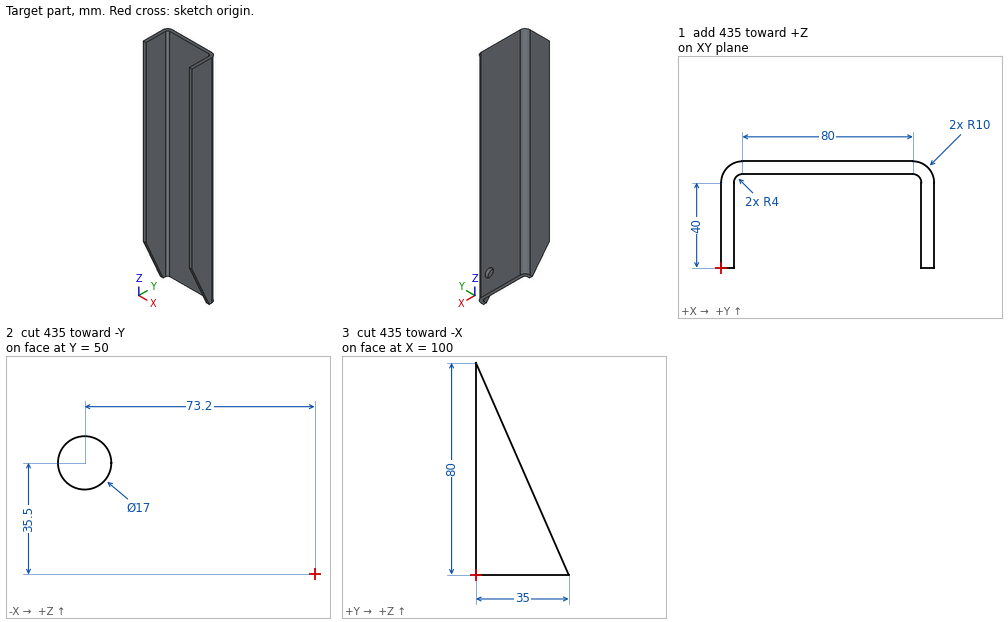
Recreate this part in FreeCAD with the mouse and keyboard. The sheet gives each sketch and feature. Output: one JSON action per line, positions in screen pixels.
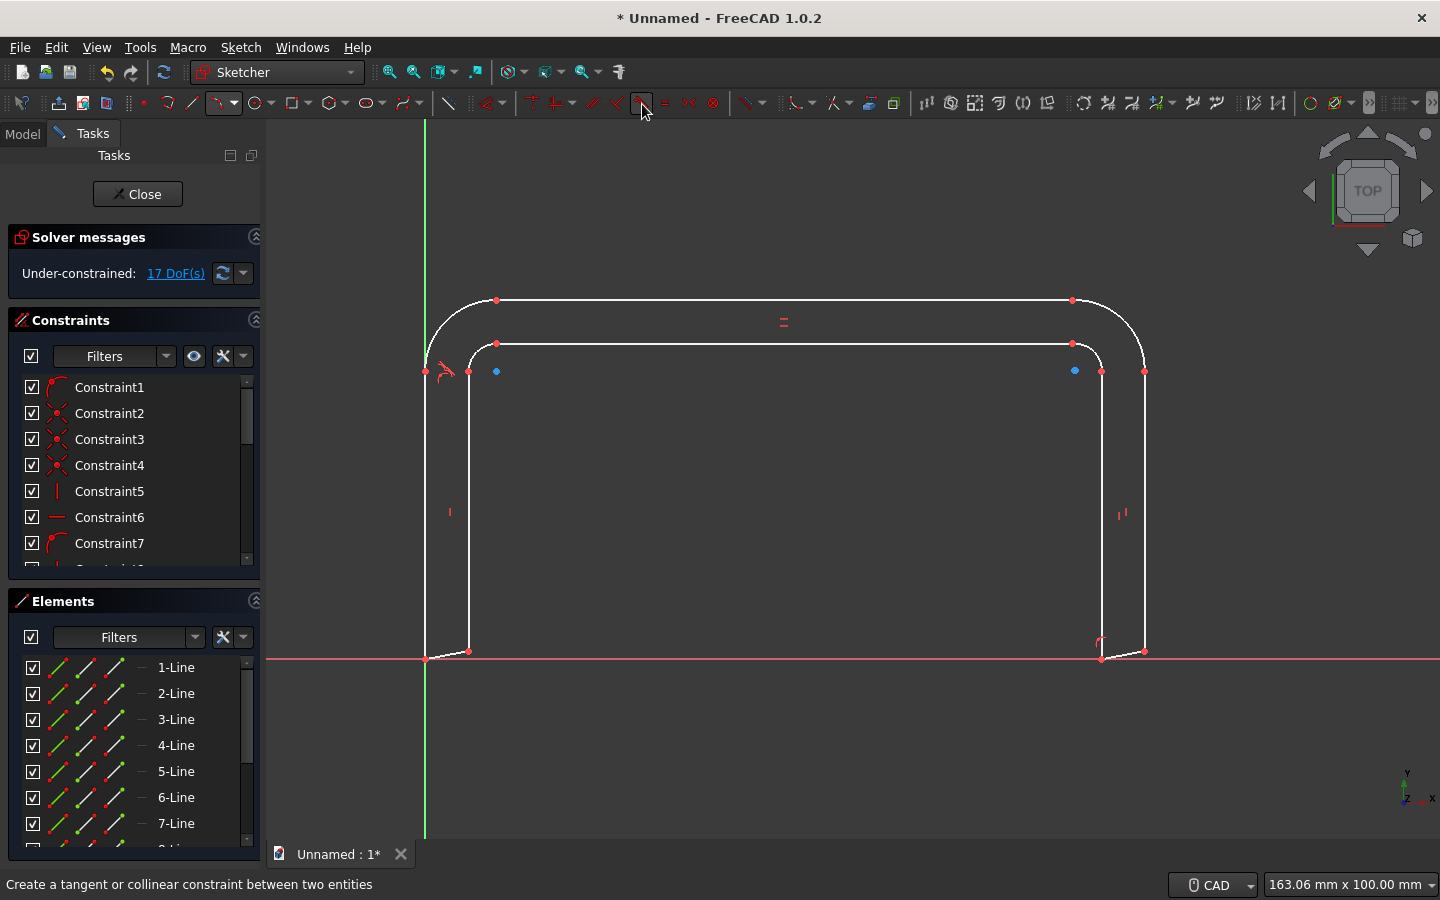
{"action": "left_click", "coordinate": [669, 344]}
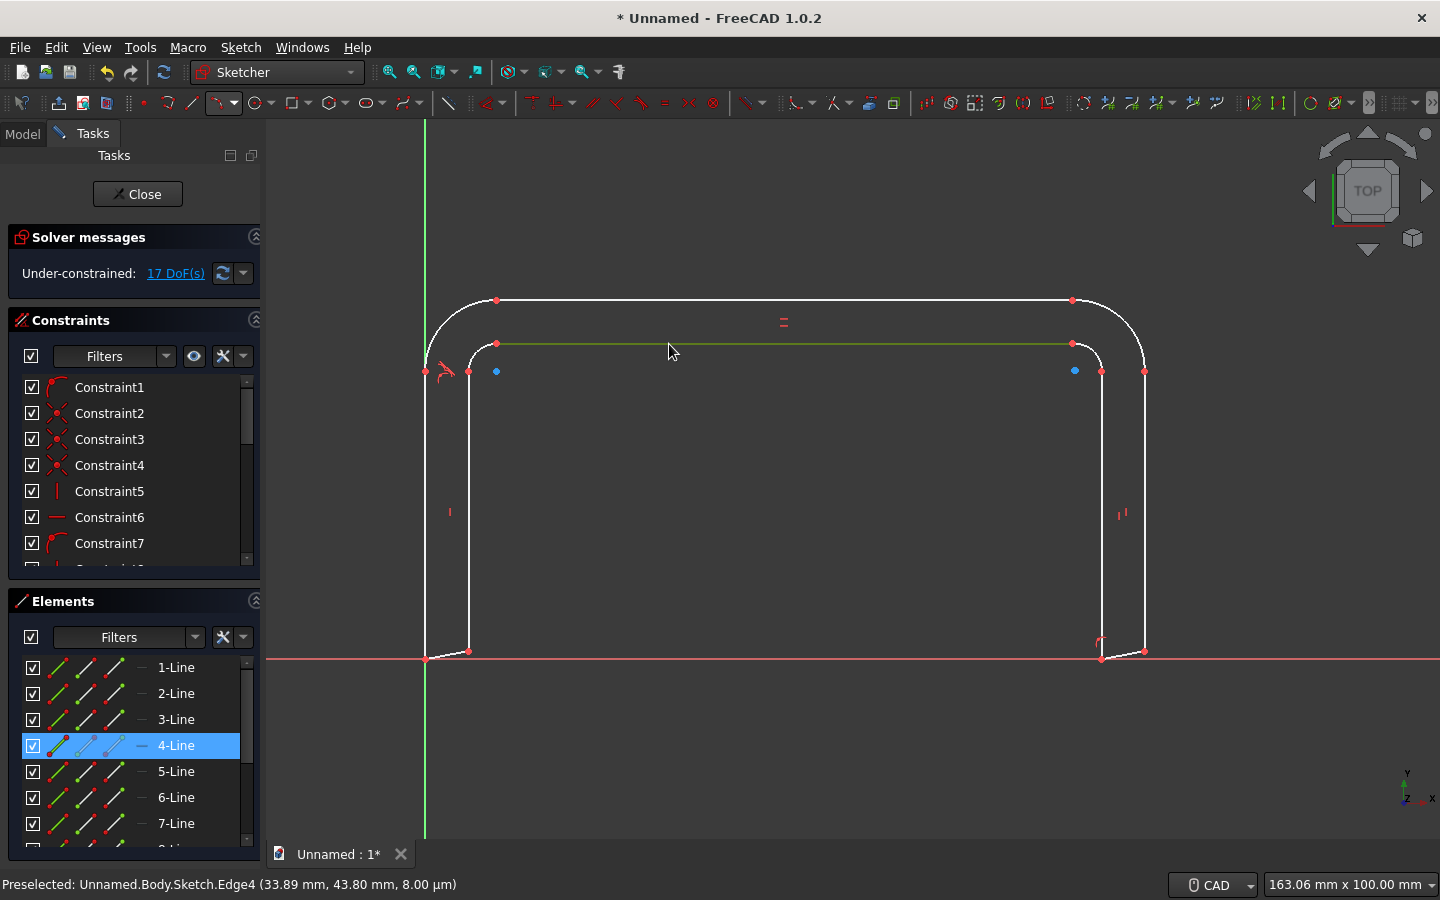
{"action": "left_click", "coordinate": [484, 347]}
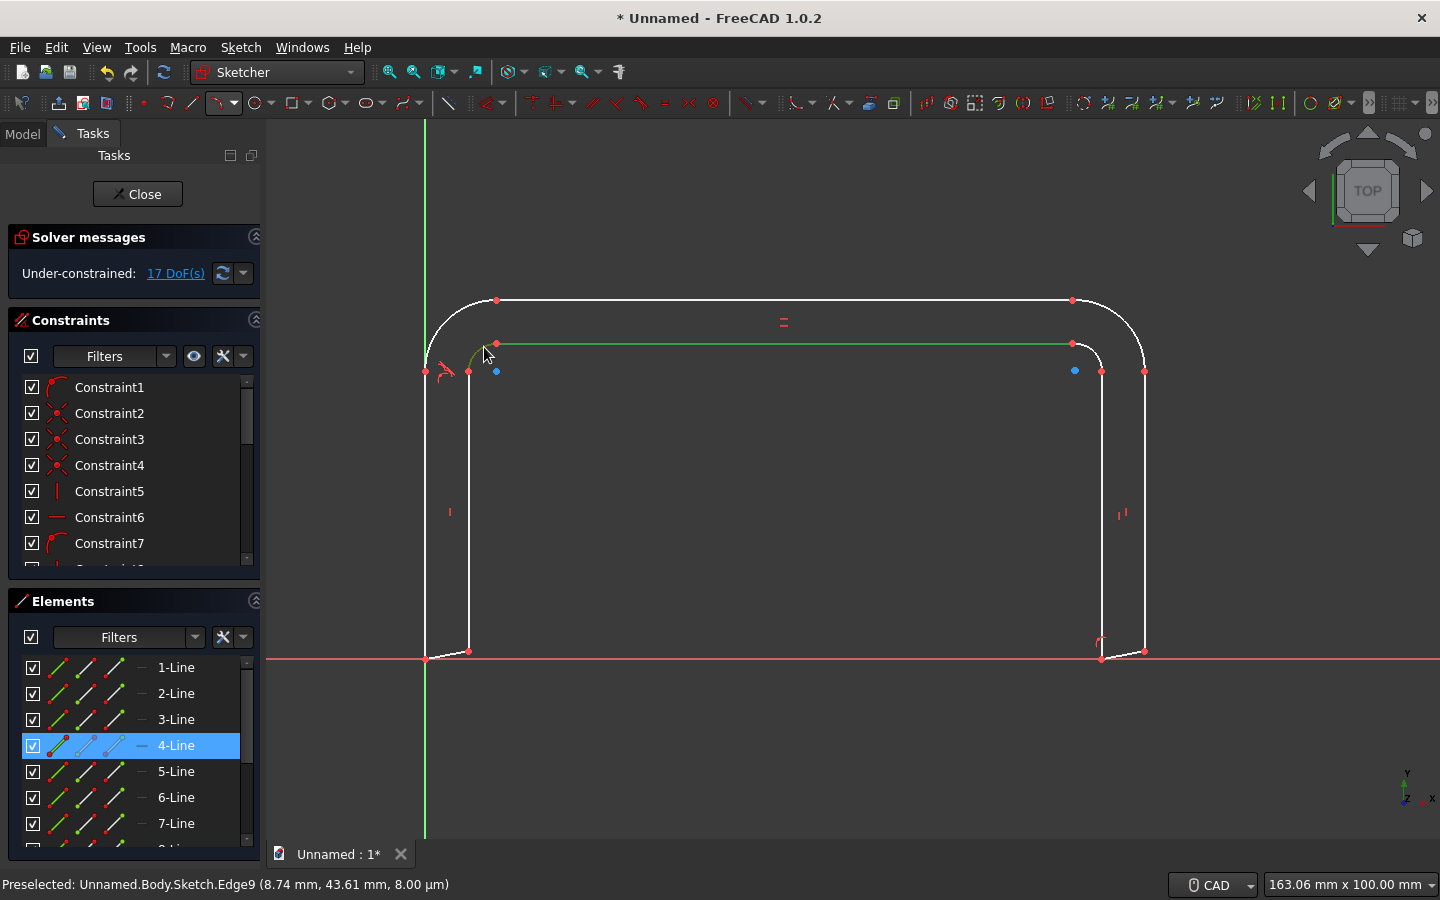
{"action": "left_click", "coordinate": [642, 104]}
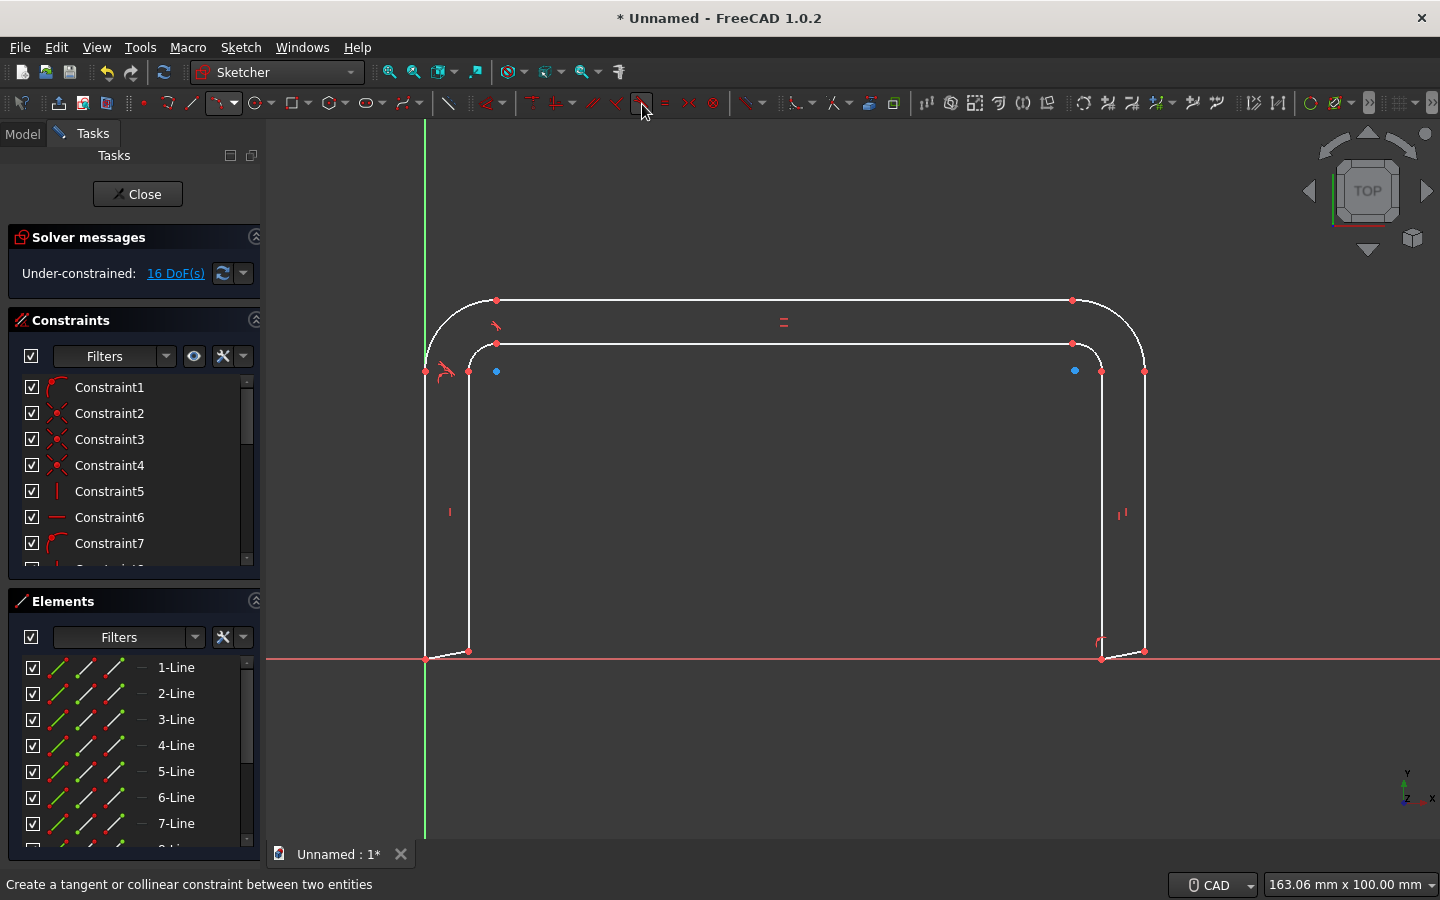
{"action": "left_click", "coordinate": [669, 344]}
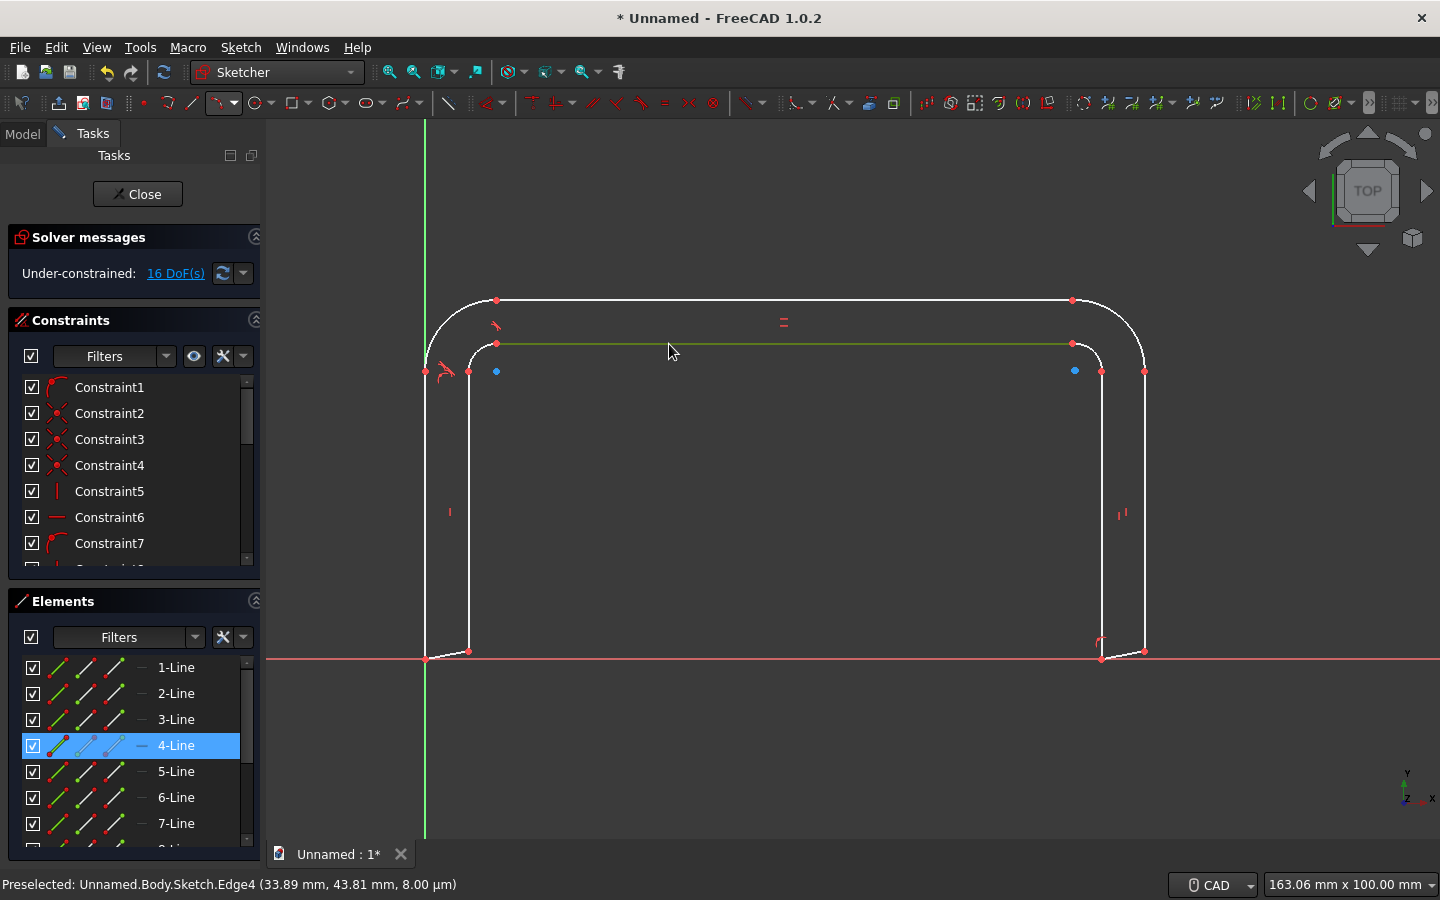
{"action": "left_click", "coordinate": [1099, 359]}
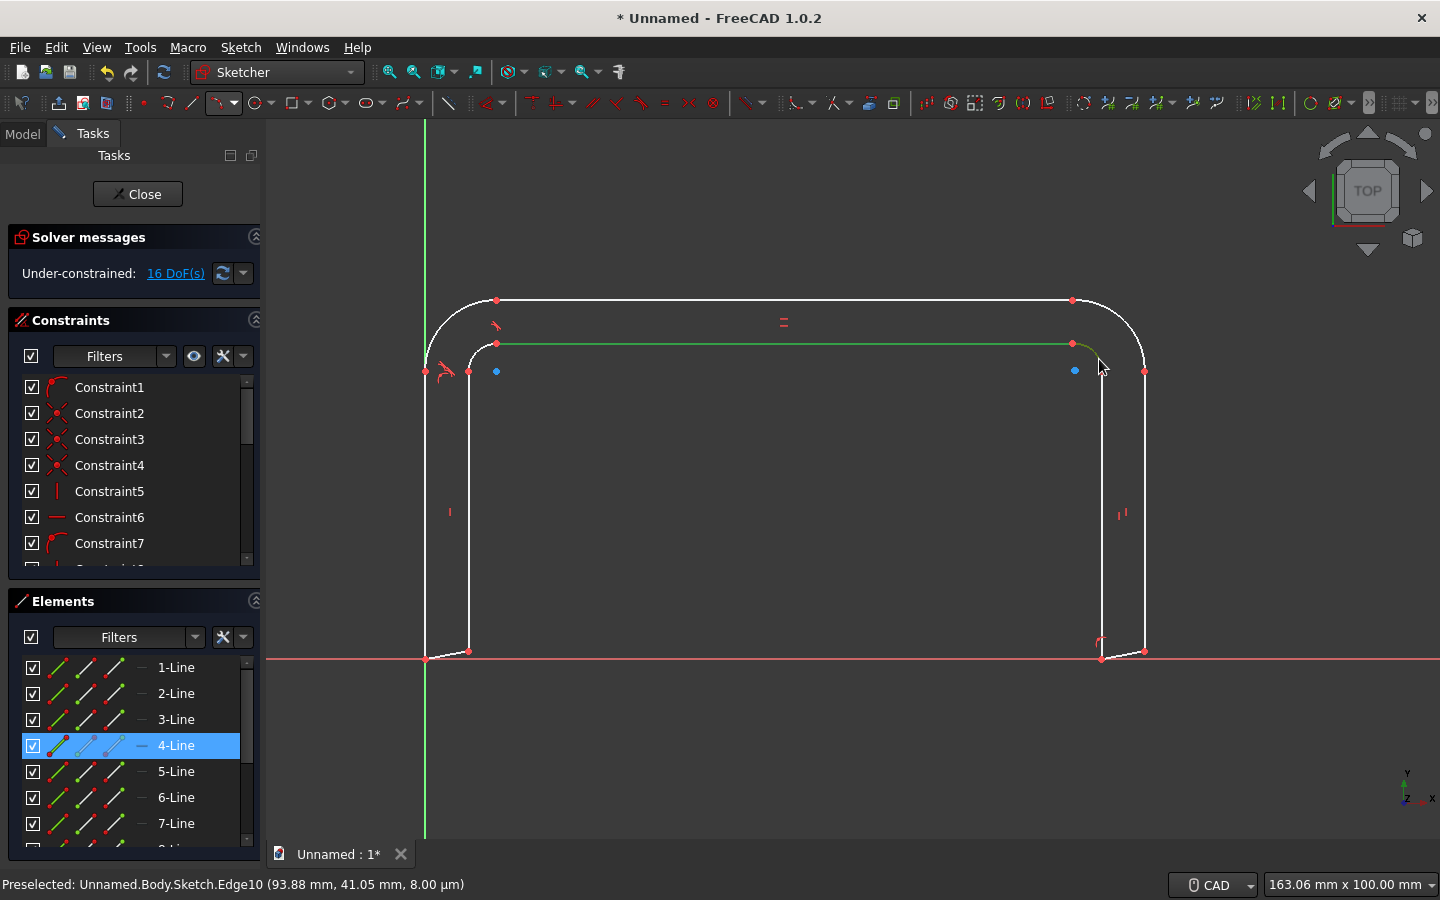
{"action": "left_click", "coordinate": [642, 104]}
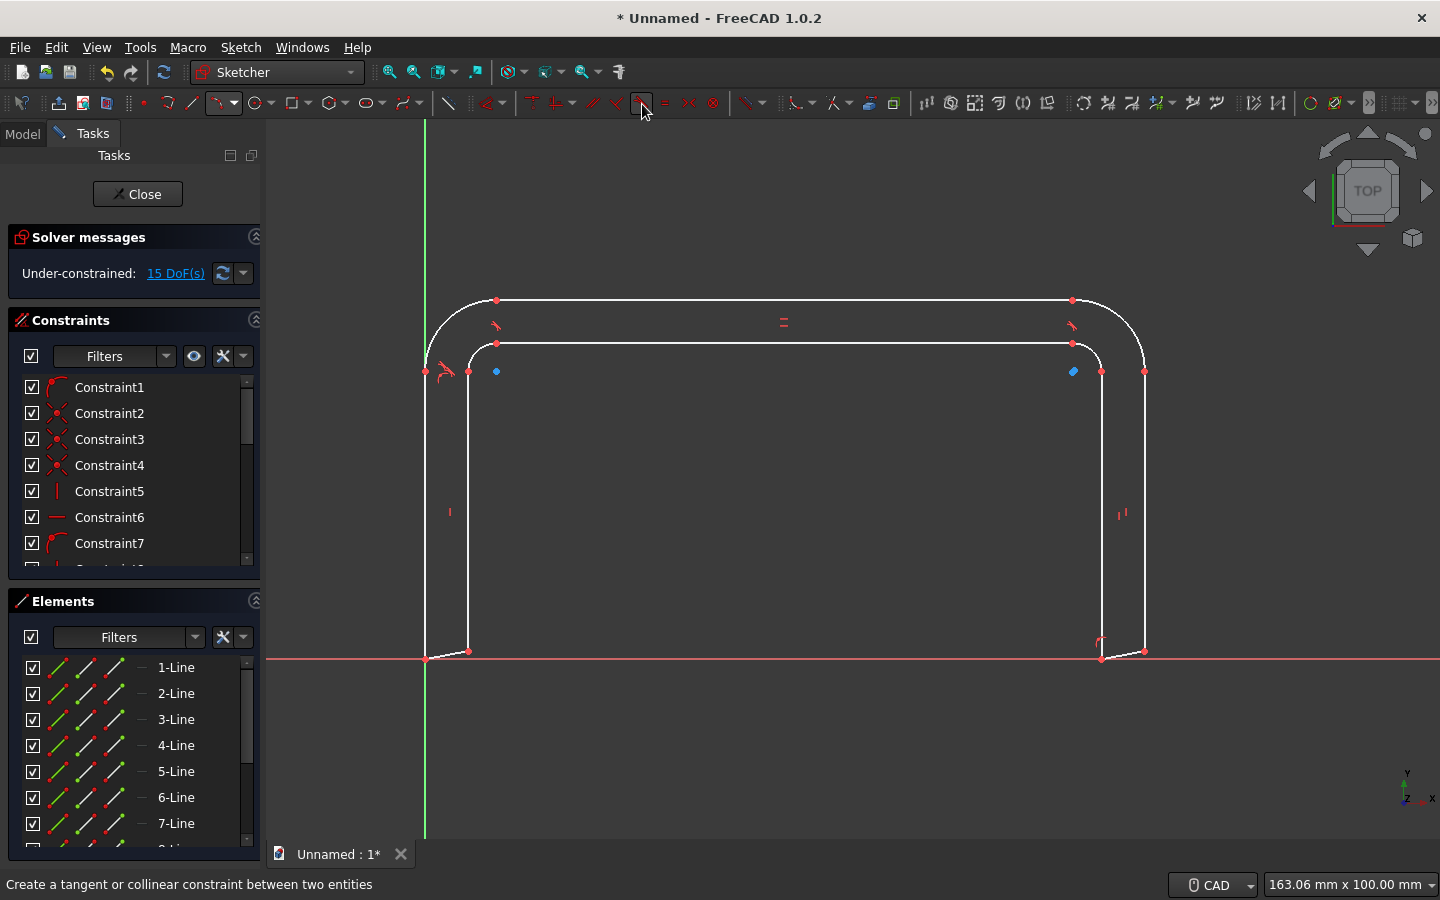
{"action": "left_click", "coordinate": [1102, 458]}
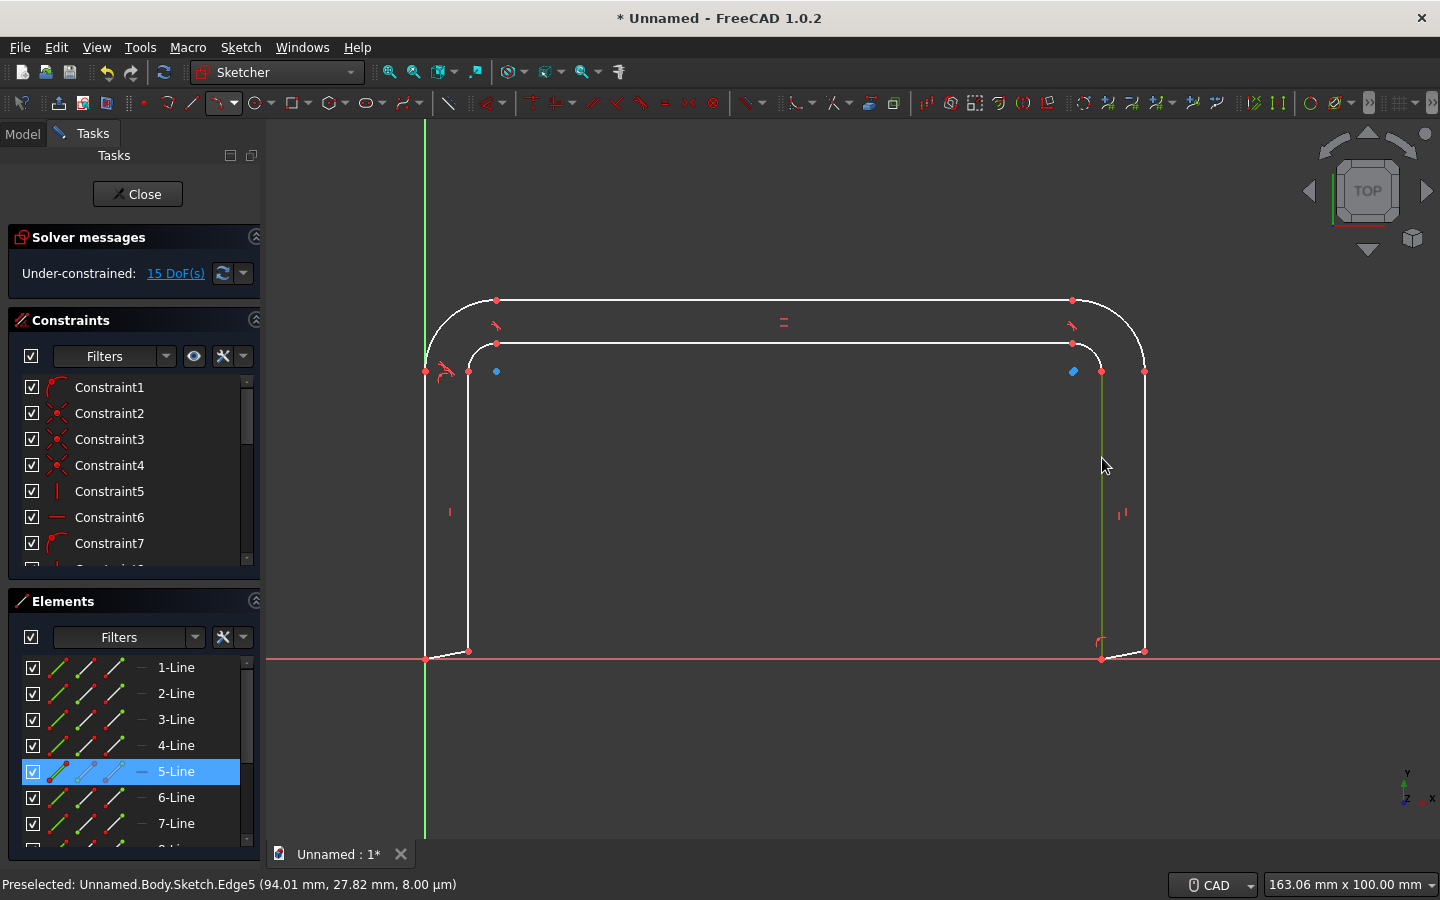
{"action": "left_click", "coordinate": [1099, 359]}